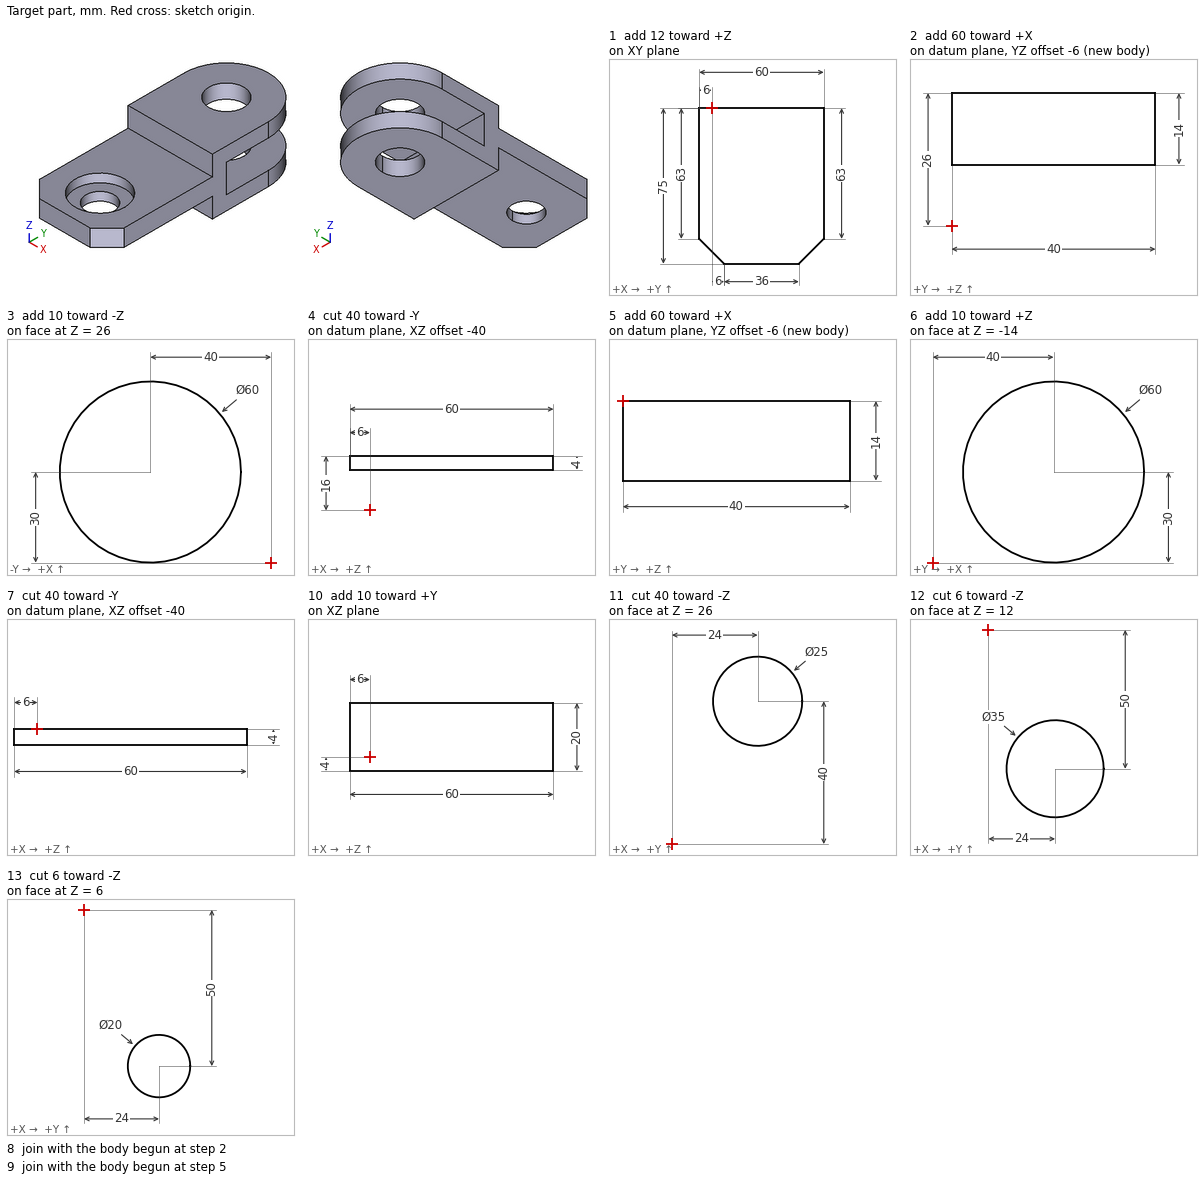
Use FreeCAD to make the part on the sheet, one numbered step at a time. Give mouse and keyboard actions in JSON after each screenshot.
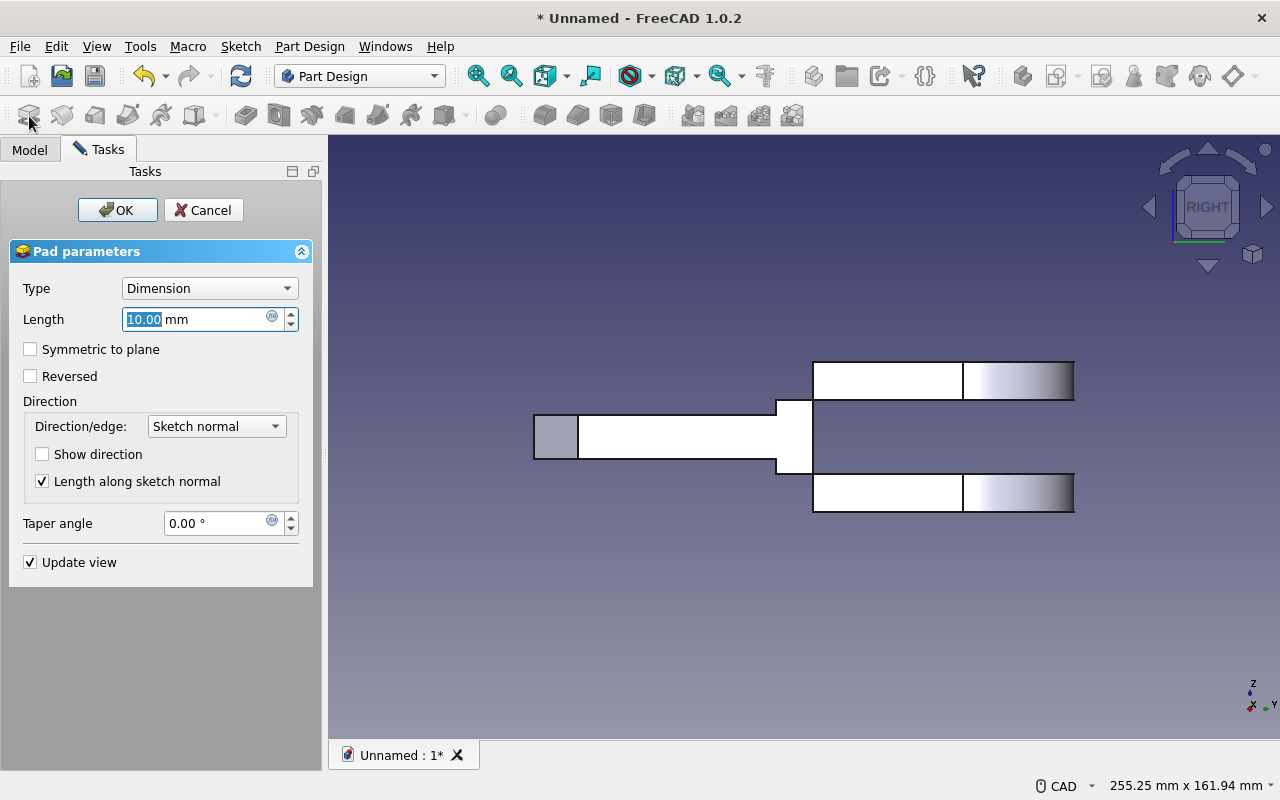
{"action": "type", "text": "10"}
{"action": "key", "text": "Tab"}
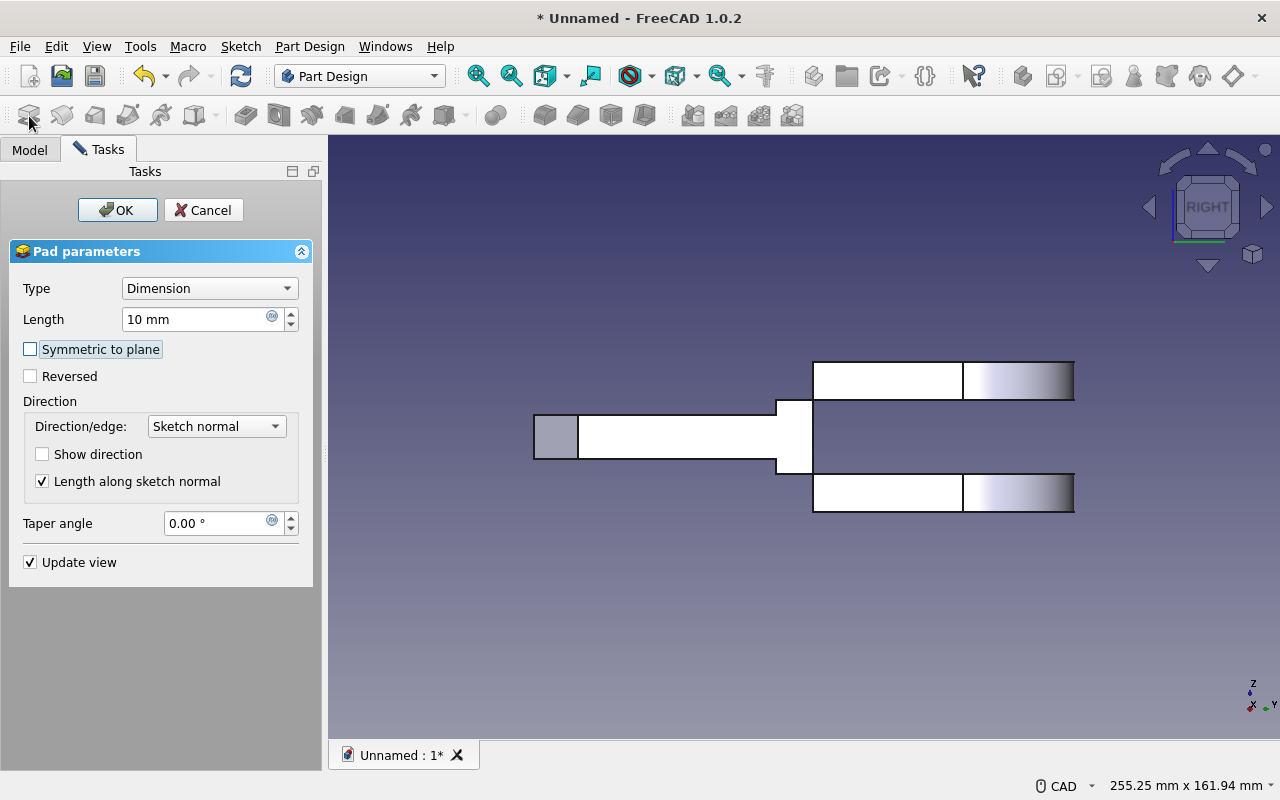
{"action": "left_click", "coordinate": [31, 376]}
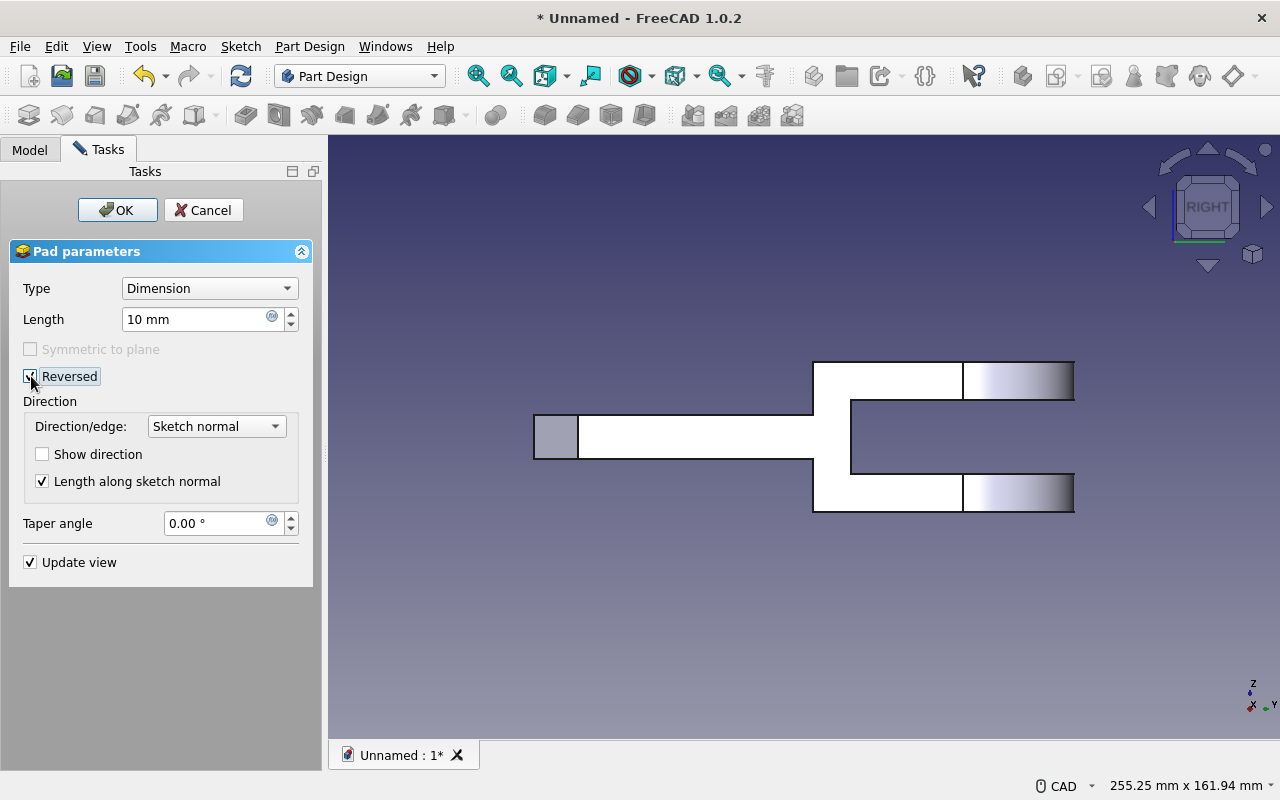
{"action": "left_click", "coordinate": [118, 210]}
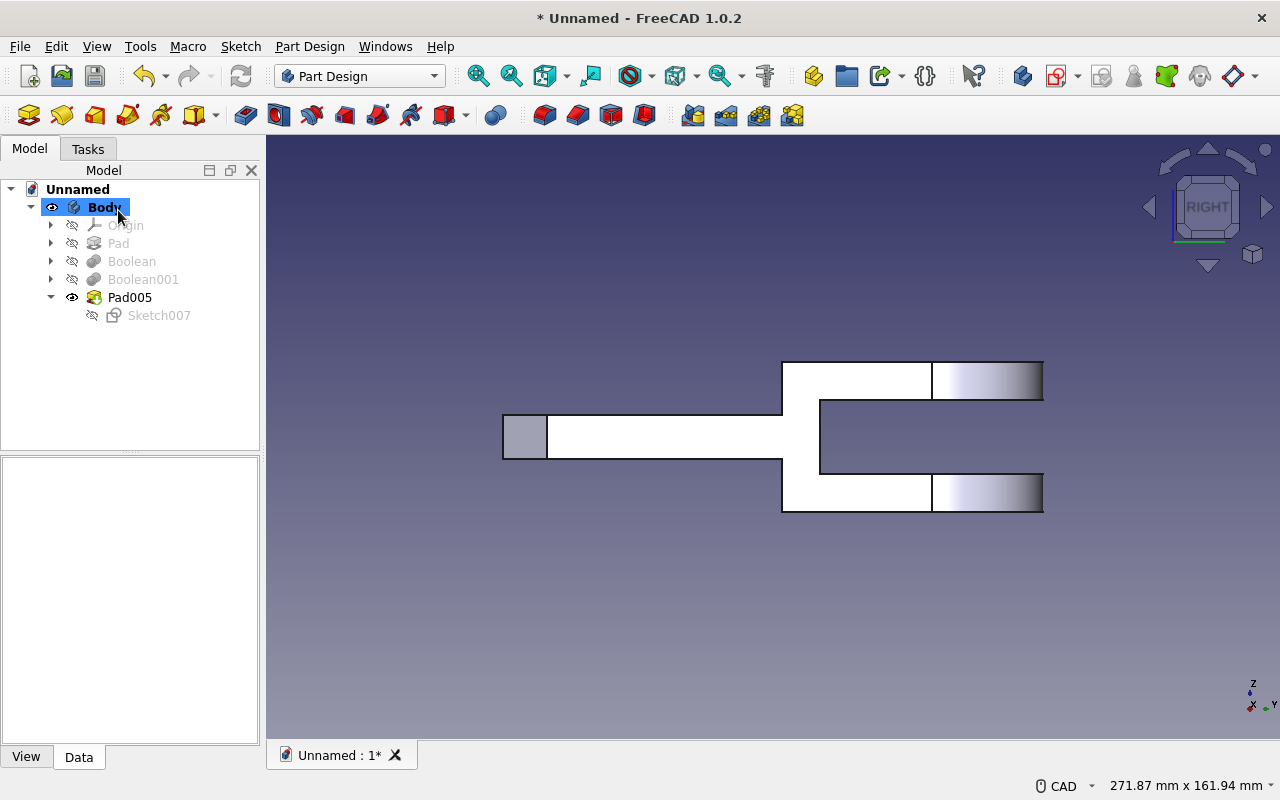
{"action": "key", "text": "0"}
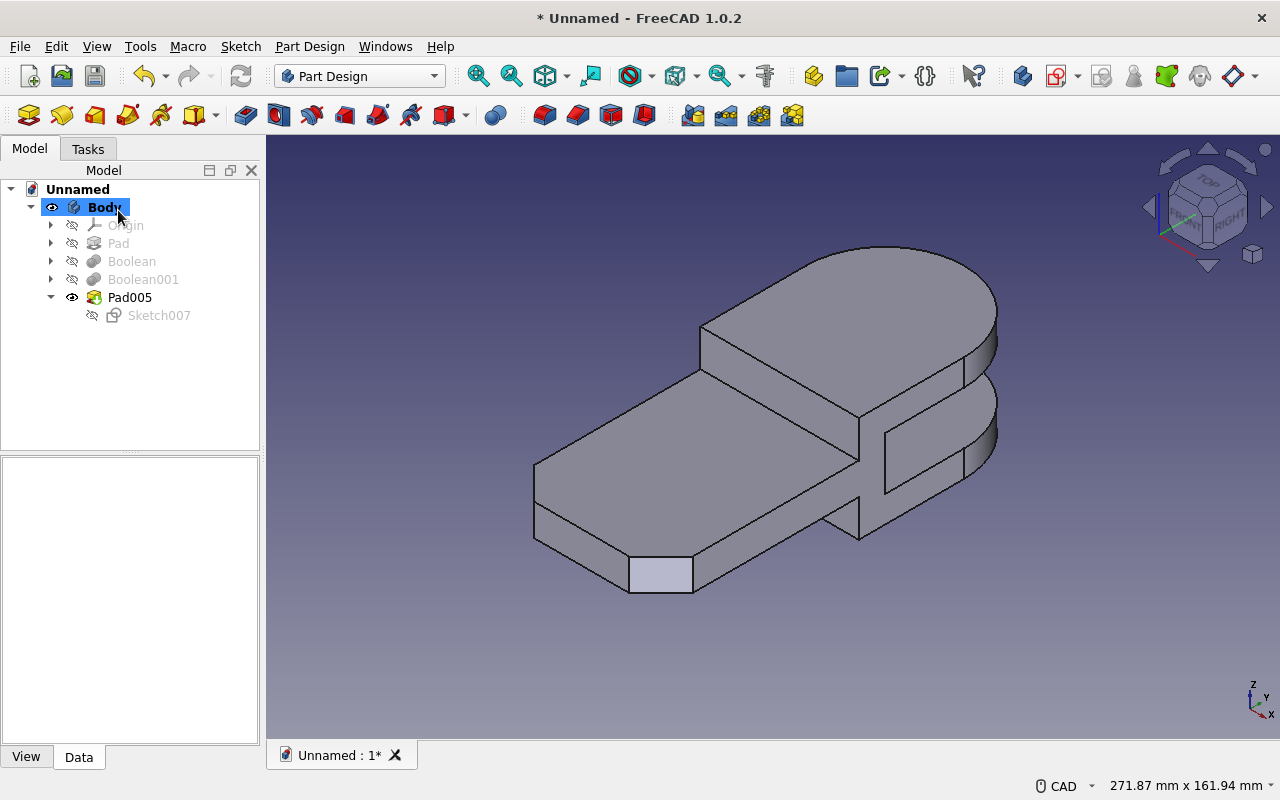
{"action": "left_click", "coordinate": [872, 318]}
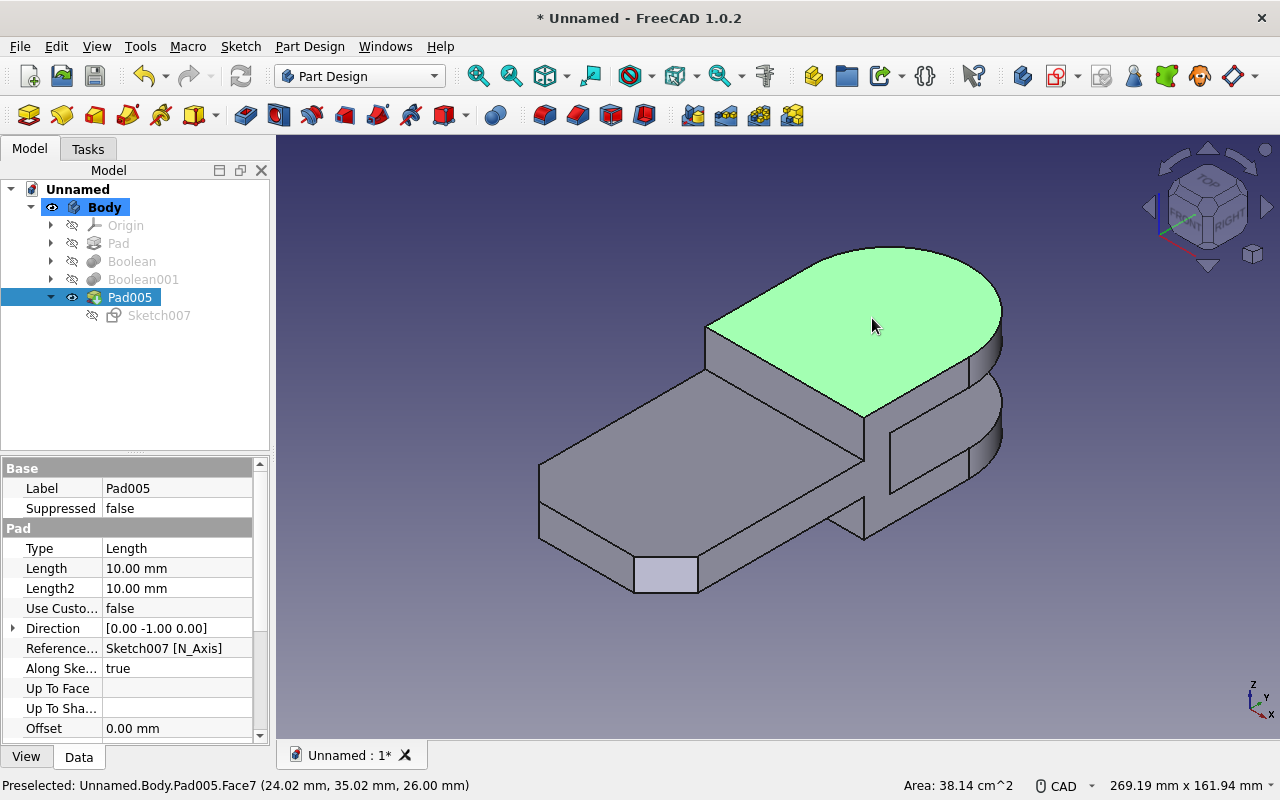
{"action": "left_click", "coordinate": [1056, 76]}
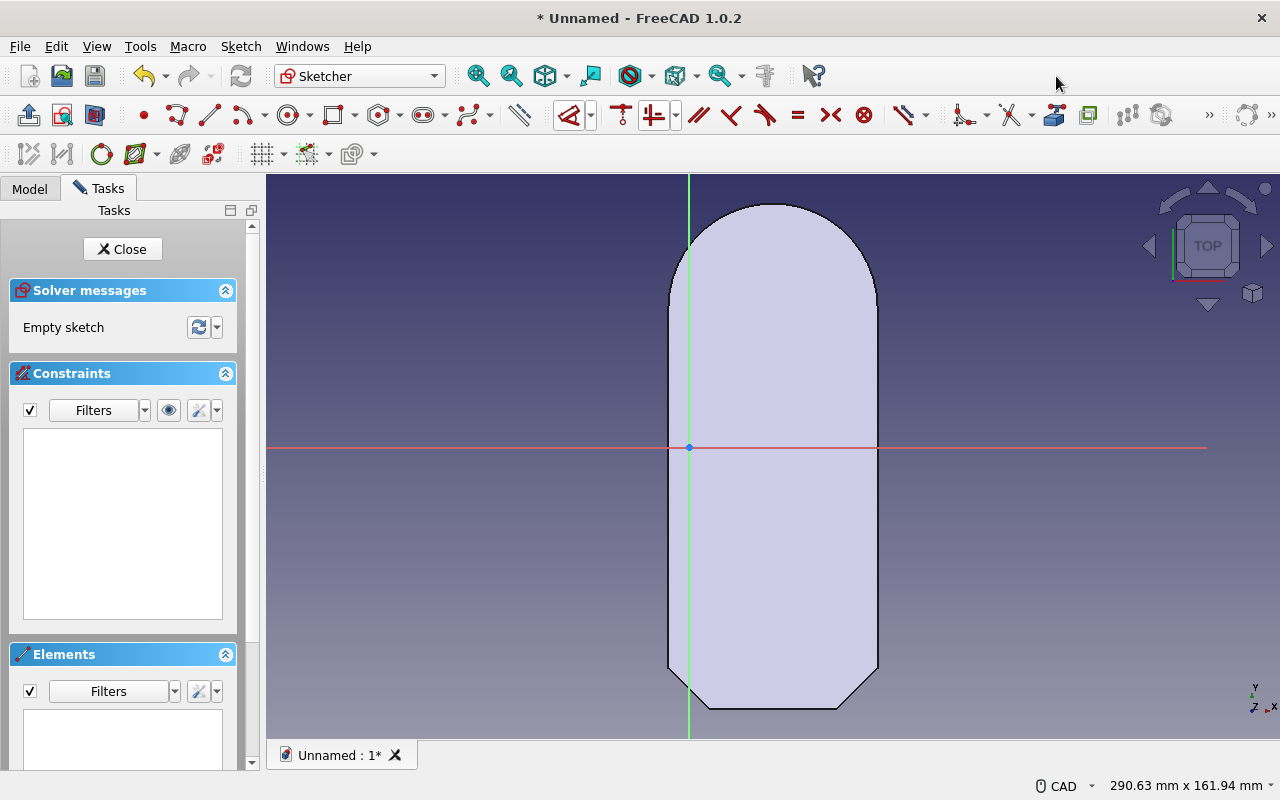
{"action": "scroll", "coordinate": [812, 234], "scroll_direction": "up", "scroll_amount": 3}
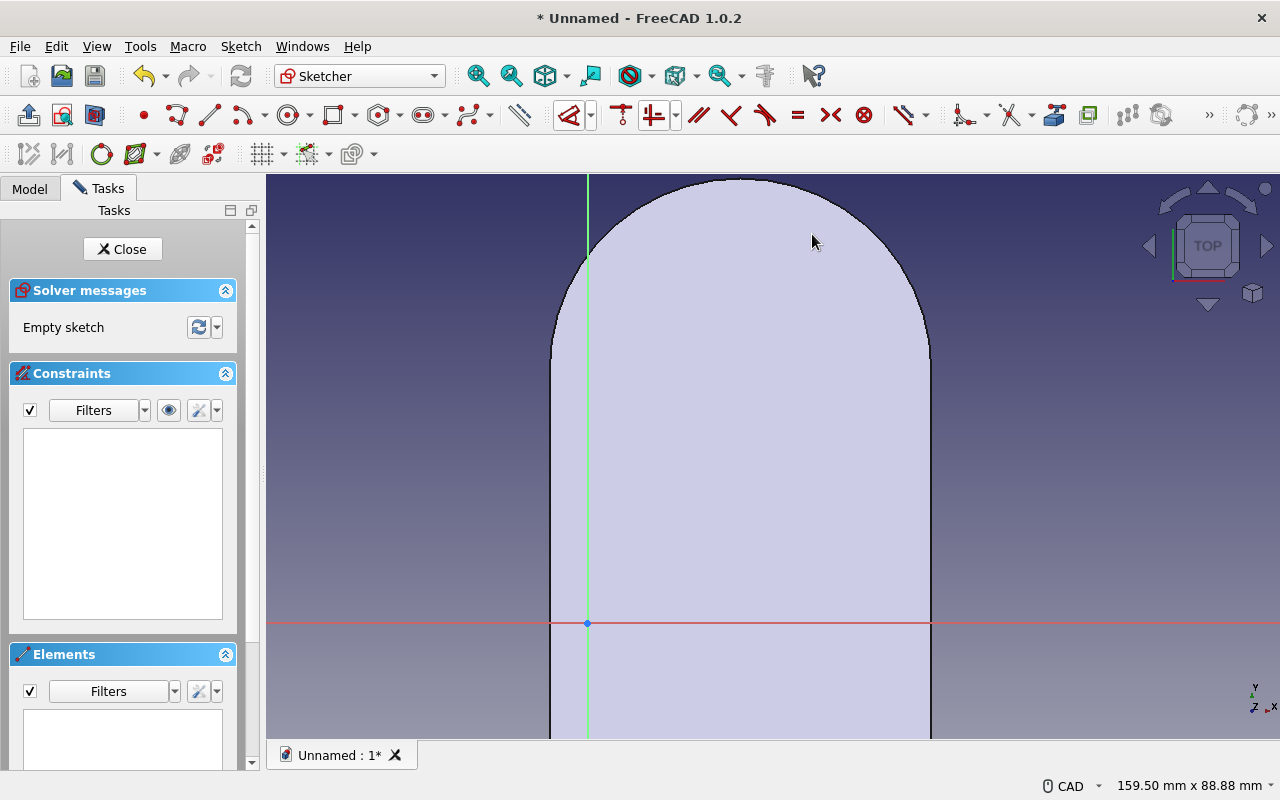
{"action": "left_click", "coordinate": [288, 116]}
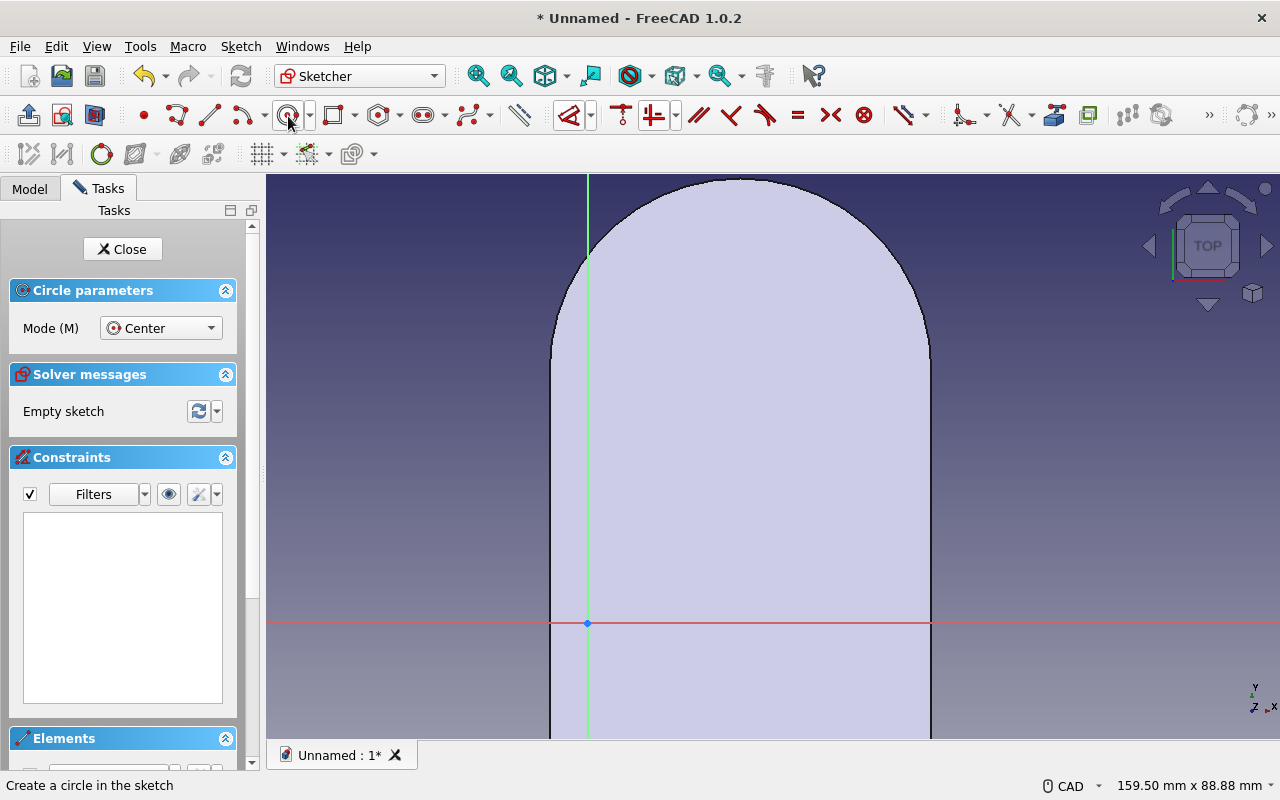
{"action": "left_click", "coordinate": [740, 369]}
{"action": "mouse_move", "coordinate": [797, 313]}